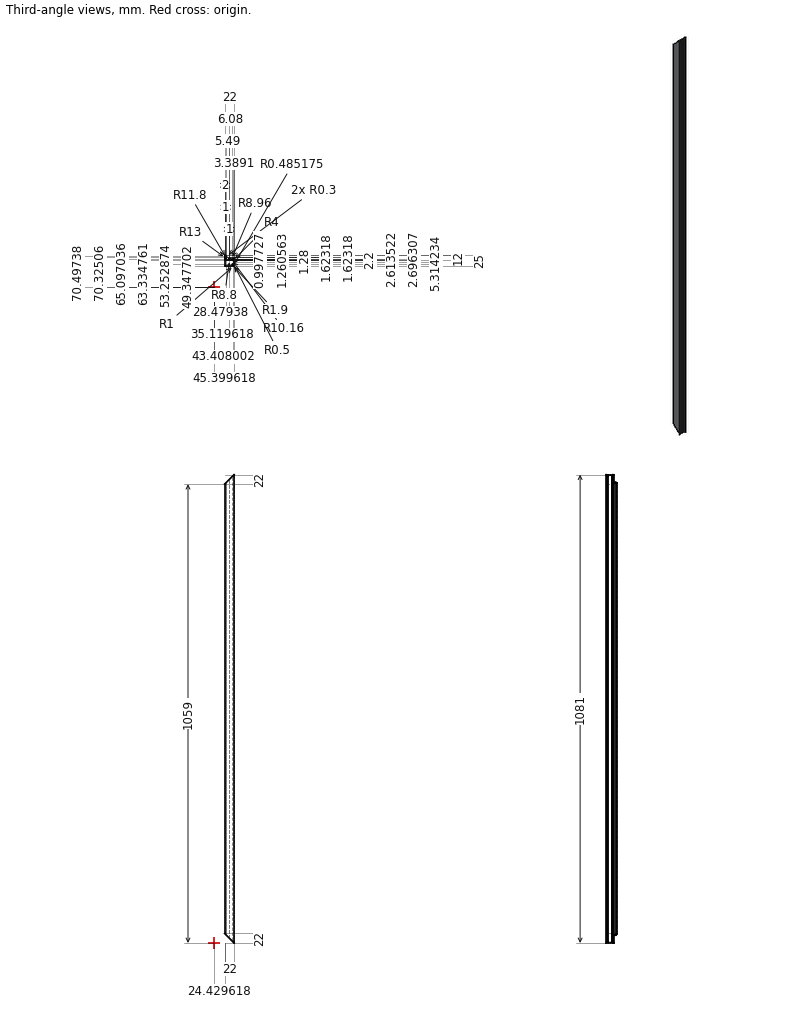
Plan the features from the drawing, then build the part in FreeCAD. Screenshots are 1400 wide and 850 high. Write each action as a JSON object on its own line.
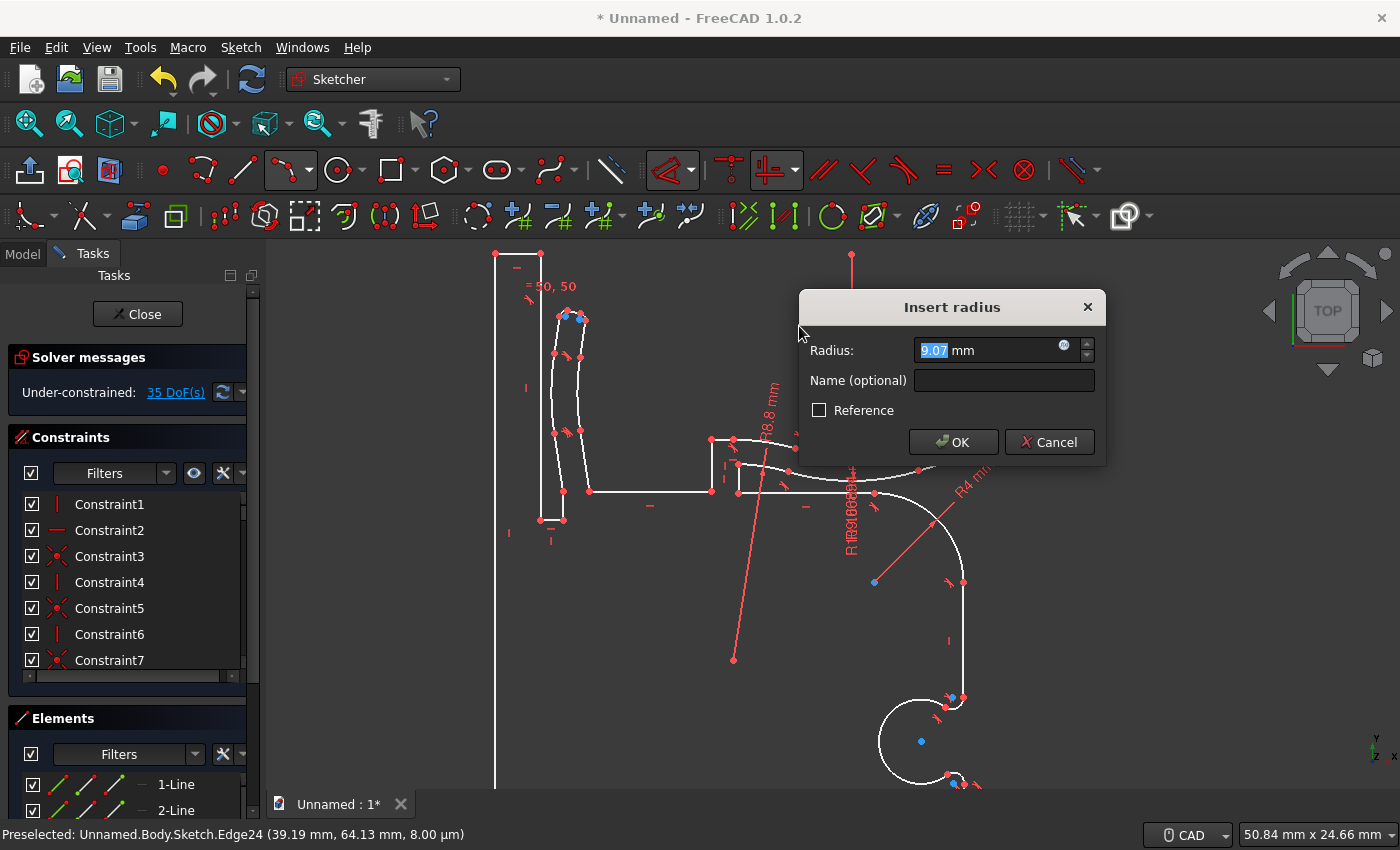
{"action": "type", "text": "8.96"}
{"action": "key", "text": "Return"}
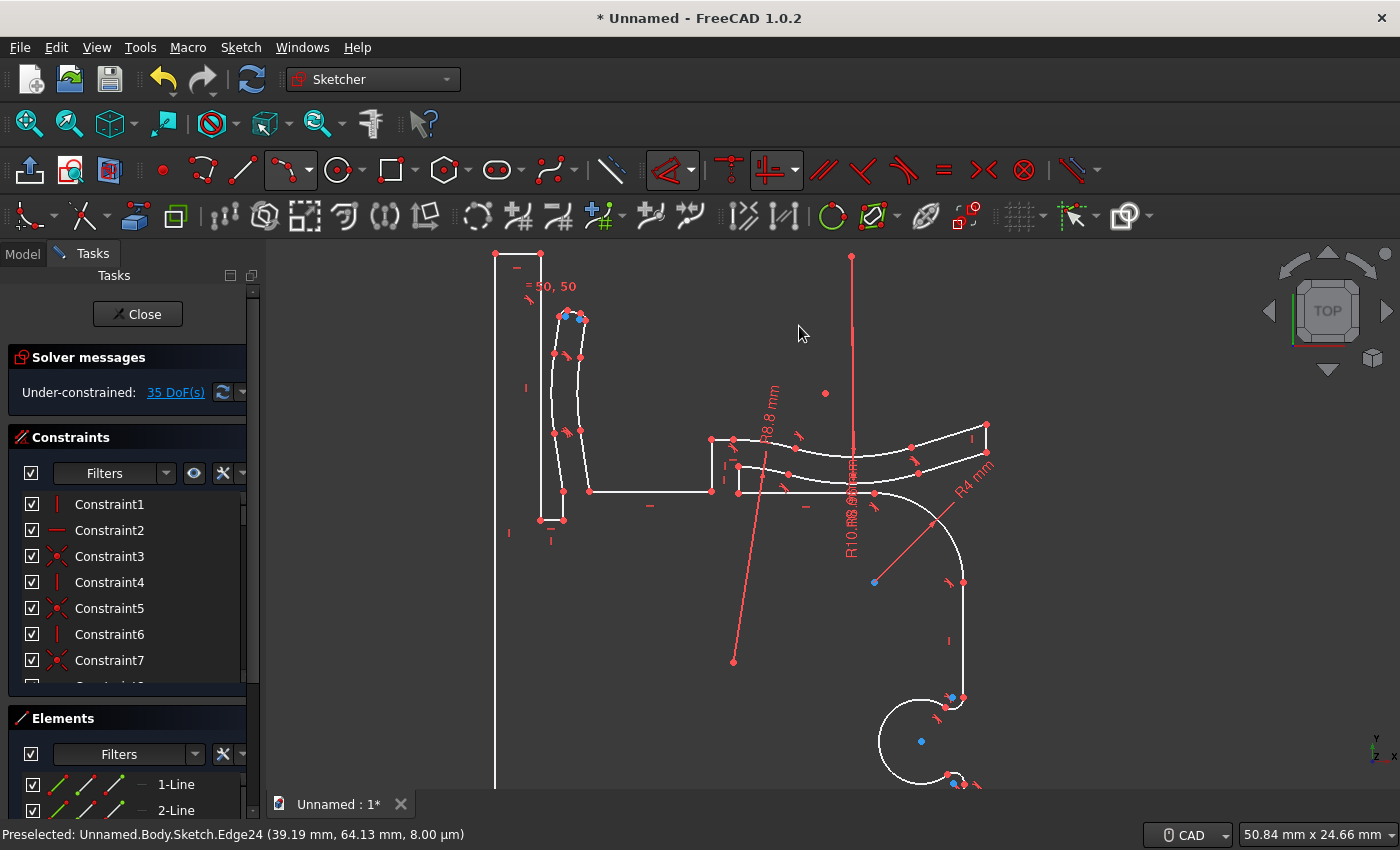
{"action": "left_click", "coordinate": [578, 379]}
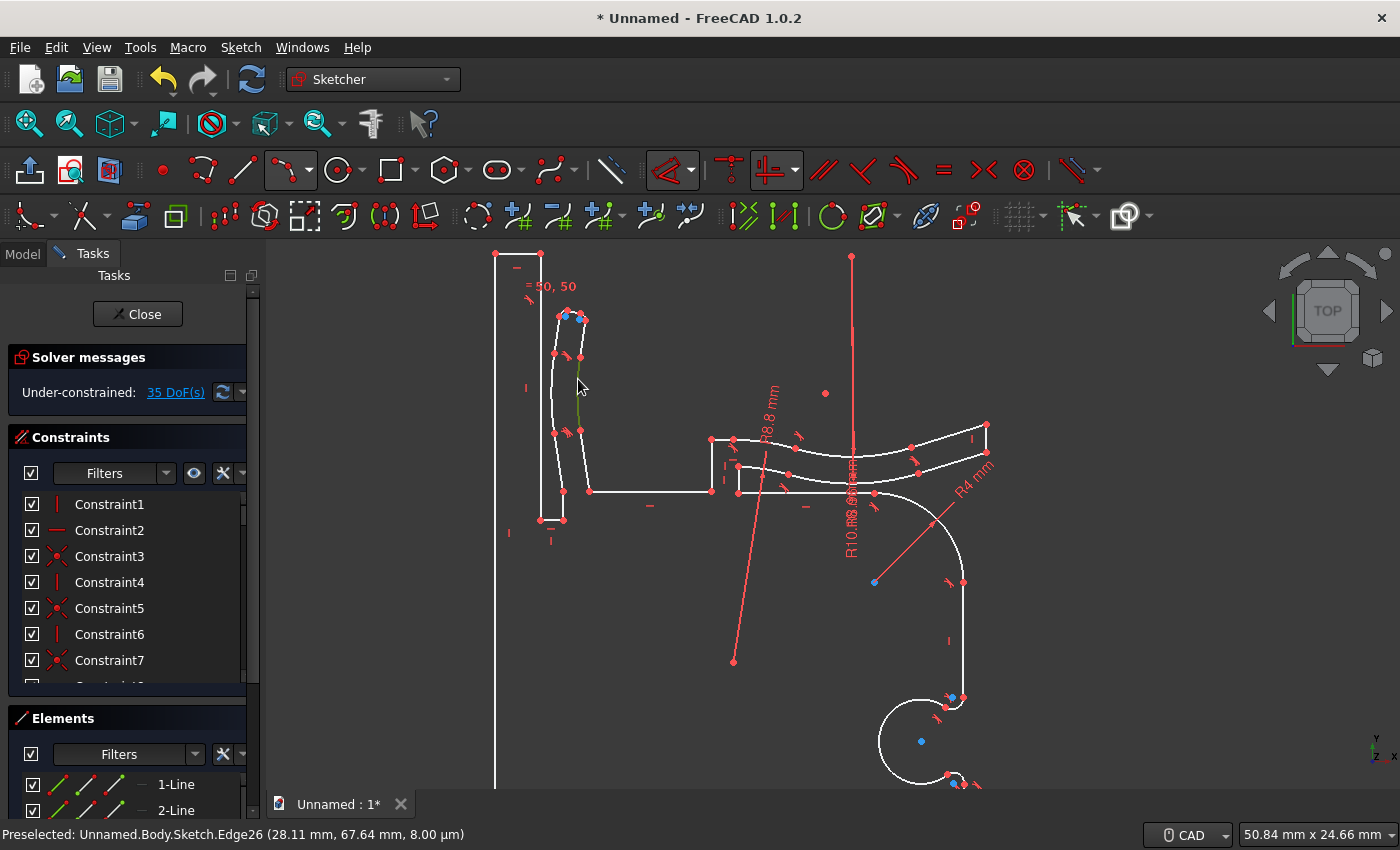
{"action": "key", "text": "k r"}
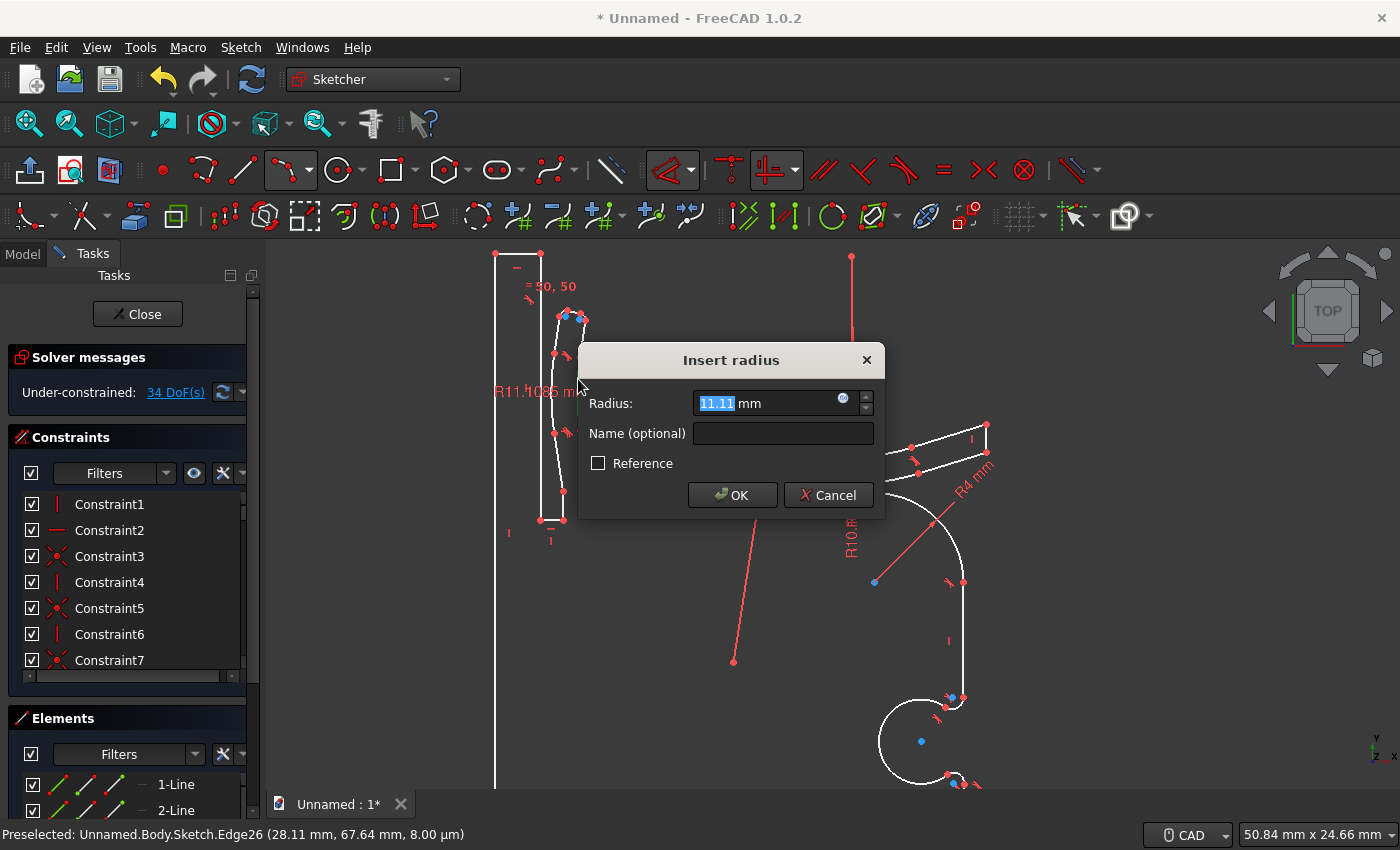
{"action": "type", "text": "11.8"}
{"action": "key", "text": "Return"}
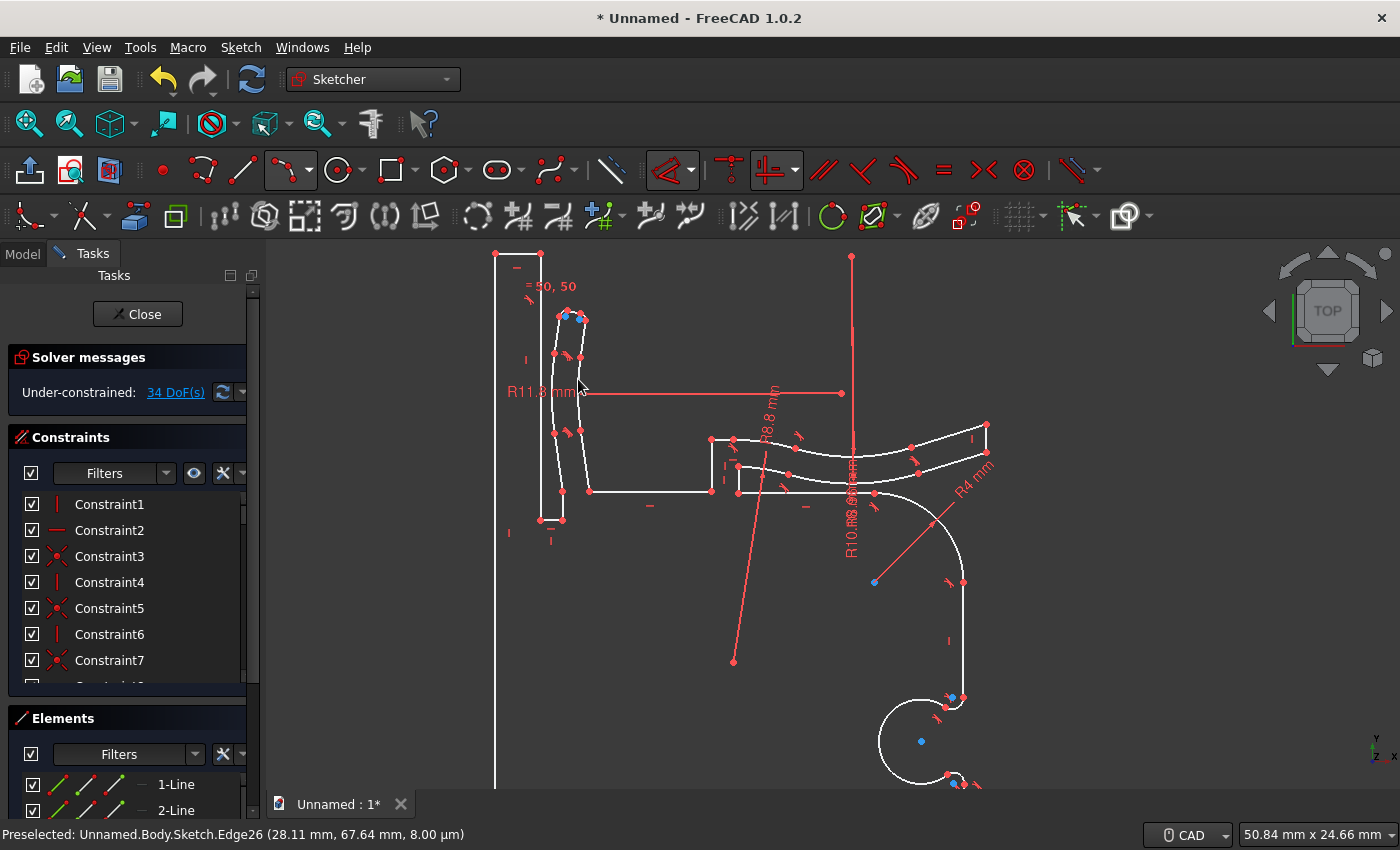
{"action": "scroll", "coordinate": [585, 316], "scroll_direction": "up", "scroll_amount": 9}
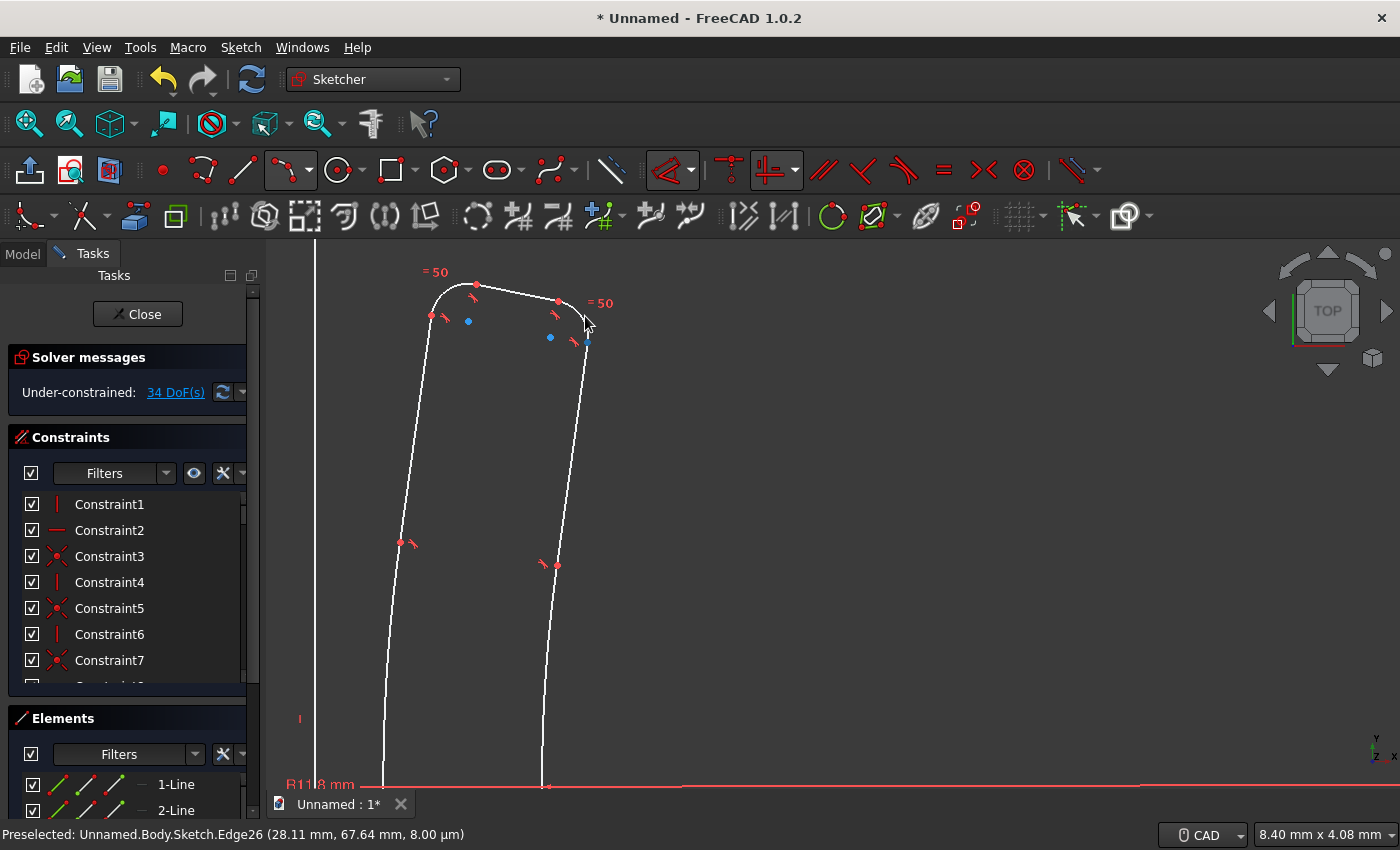
{"action": "left_click", "coordinate": [581, 316]}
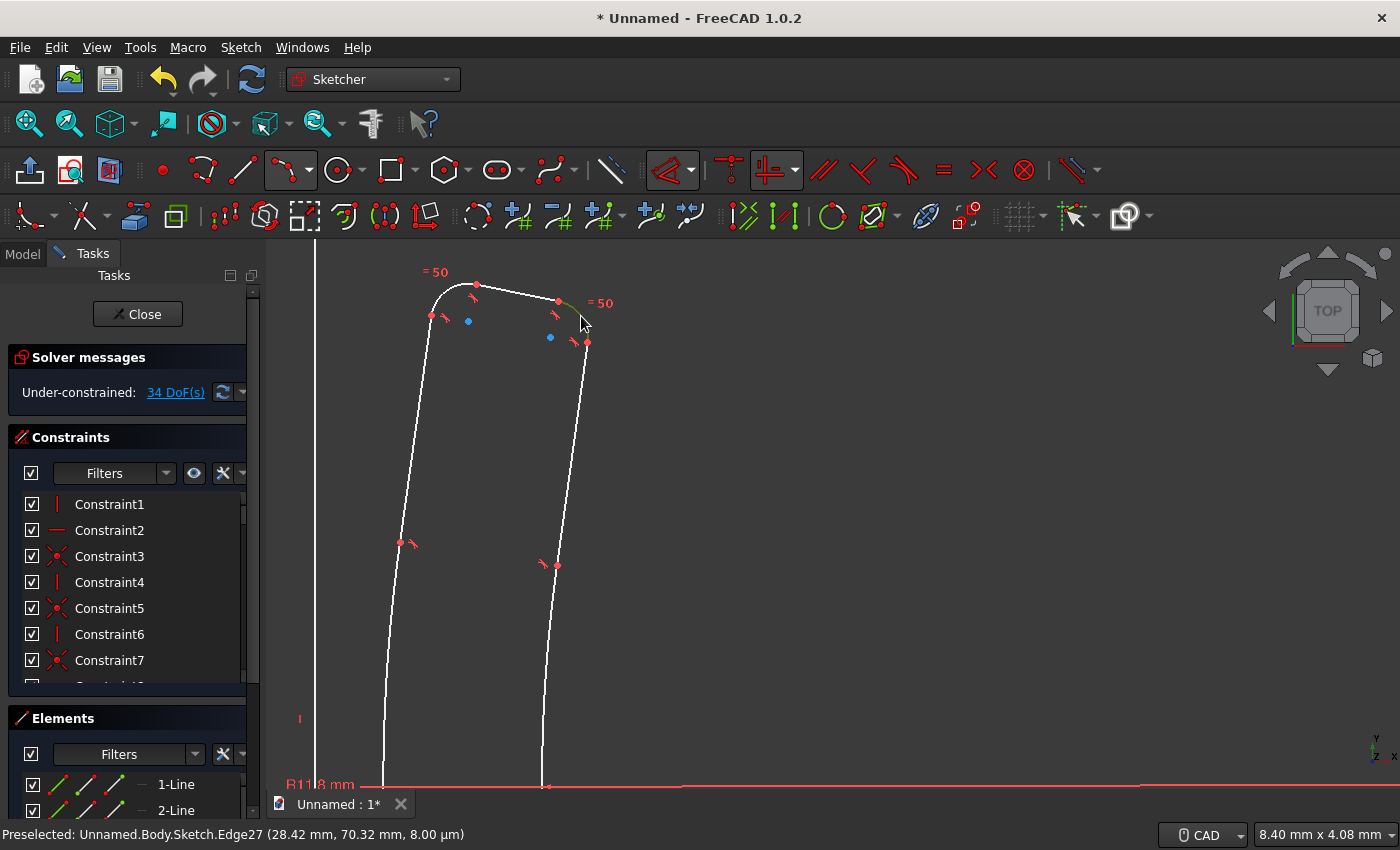
{"action": "left_click", "coordinate": [694, 170]}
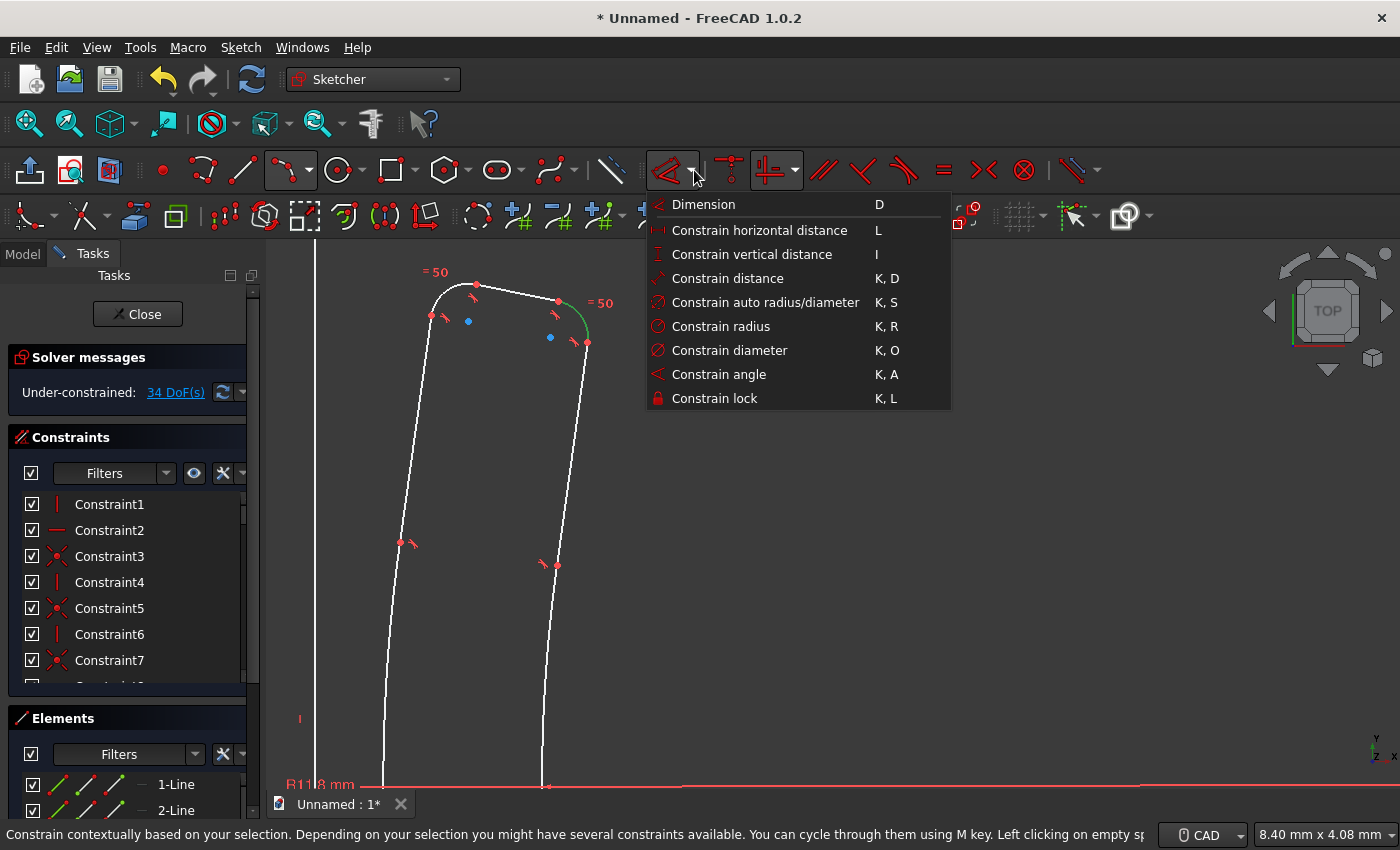
{"action": "left_click", "coordinate": [799, 326]}